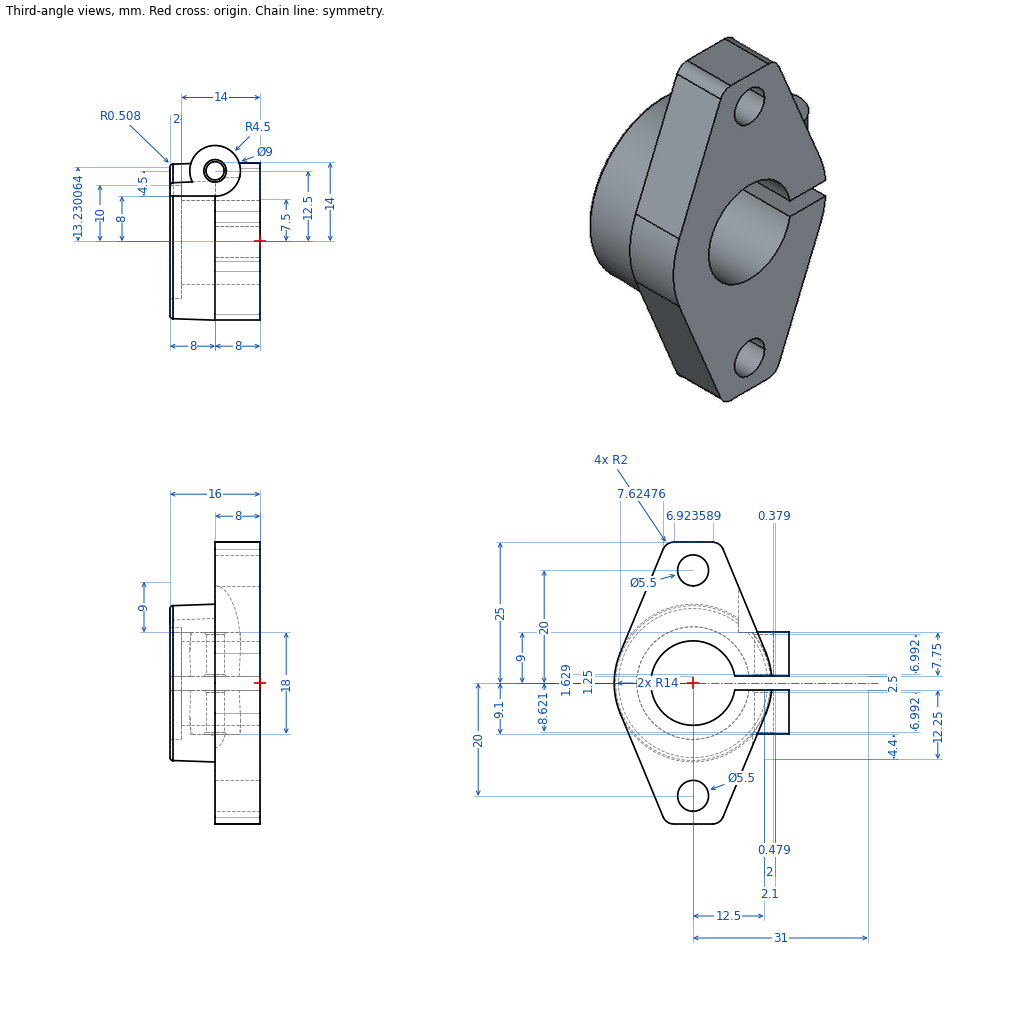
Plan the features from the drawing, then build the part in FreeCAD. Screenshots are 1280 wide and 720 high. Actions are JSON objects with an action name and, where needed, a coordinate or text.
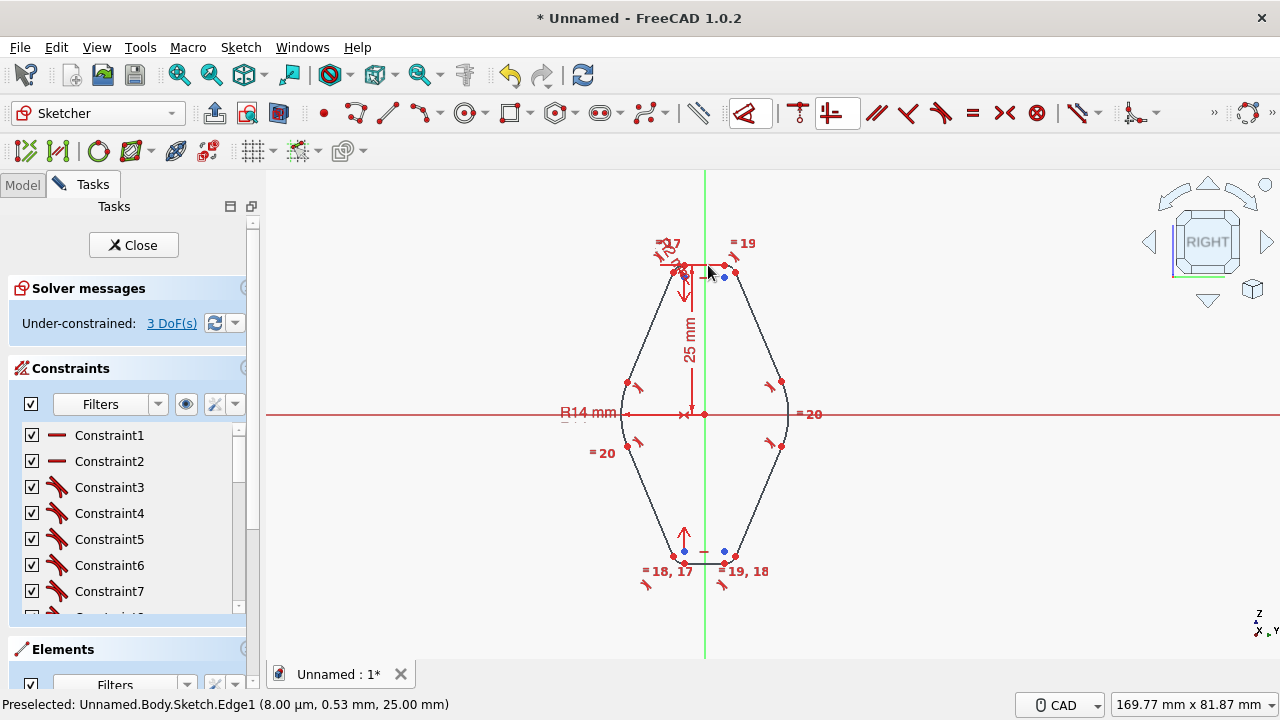
{"action": "key", "text": "l"}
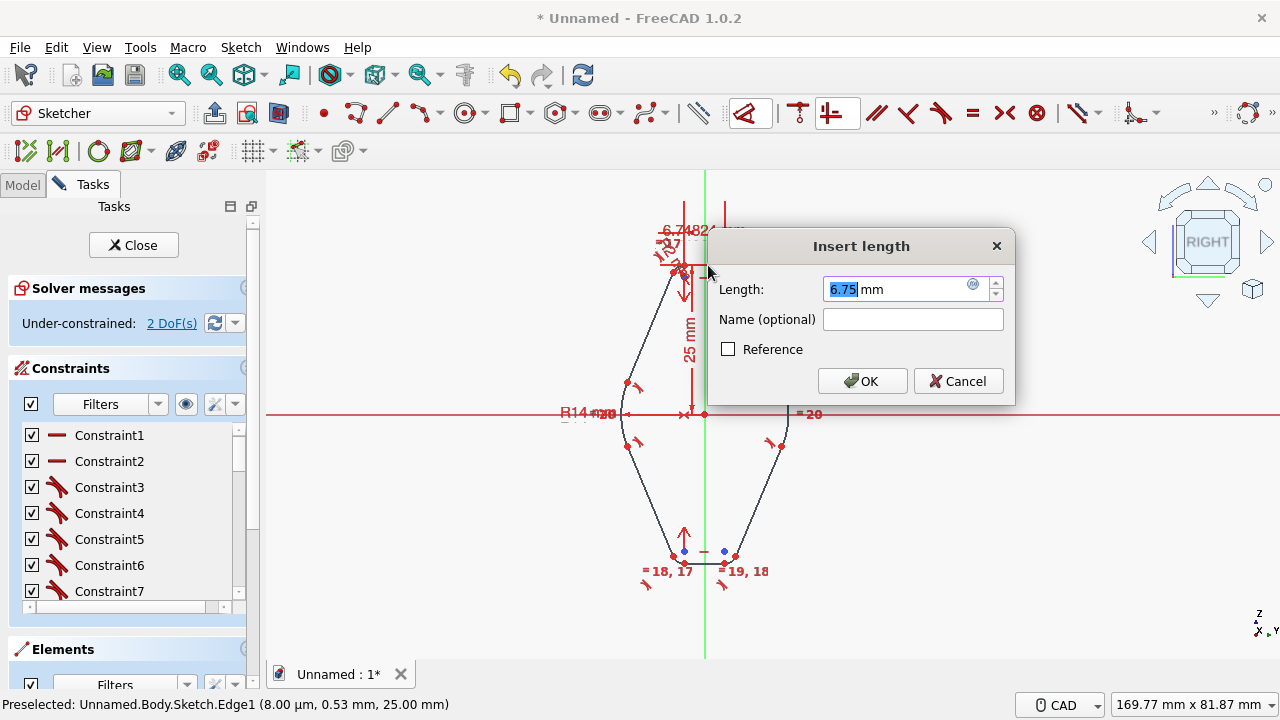
{"action": "type", "text": "6.923589"}
{"action": "key", "text": "Return"}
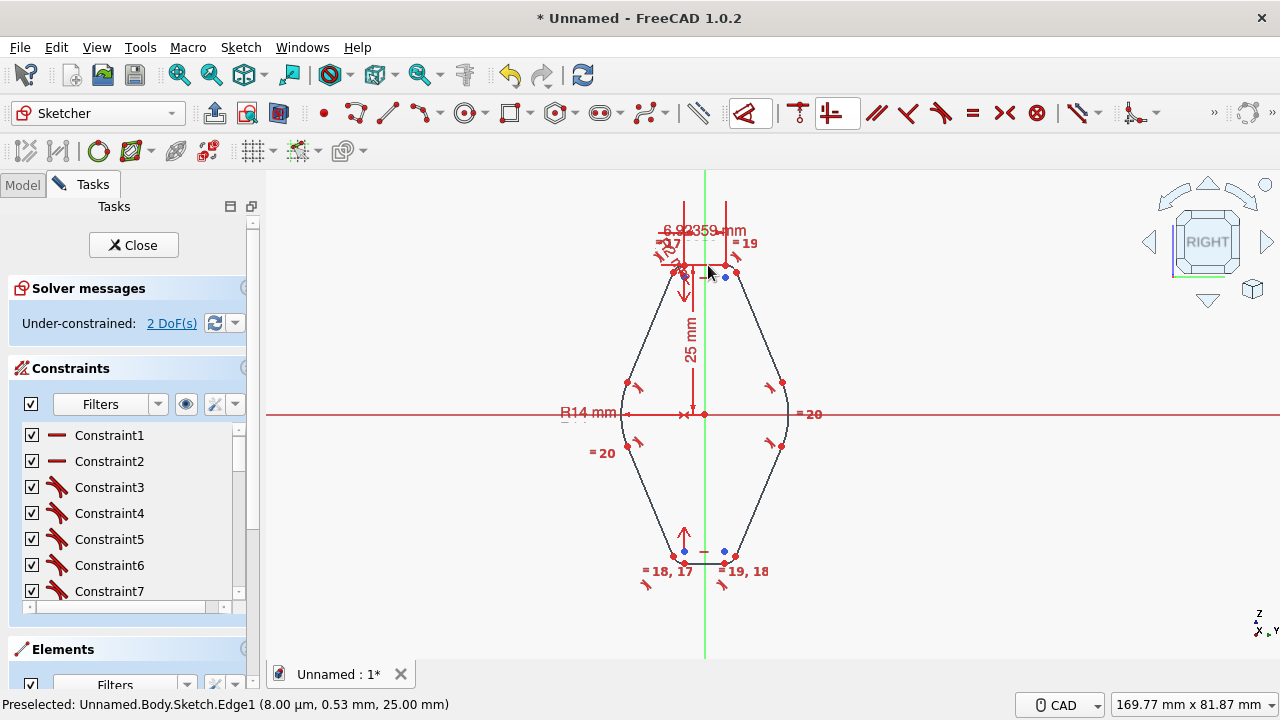
{"action": "left_click", "coordinate": [709, 564]}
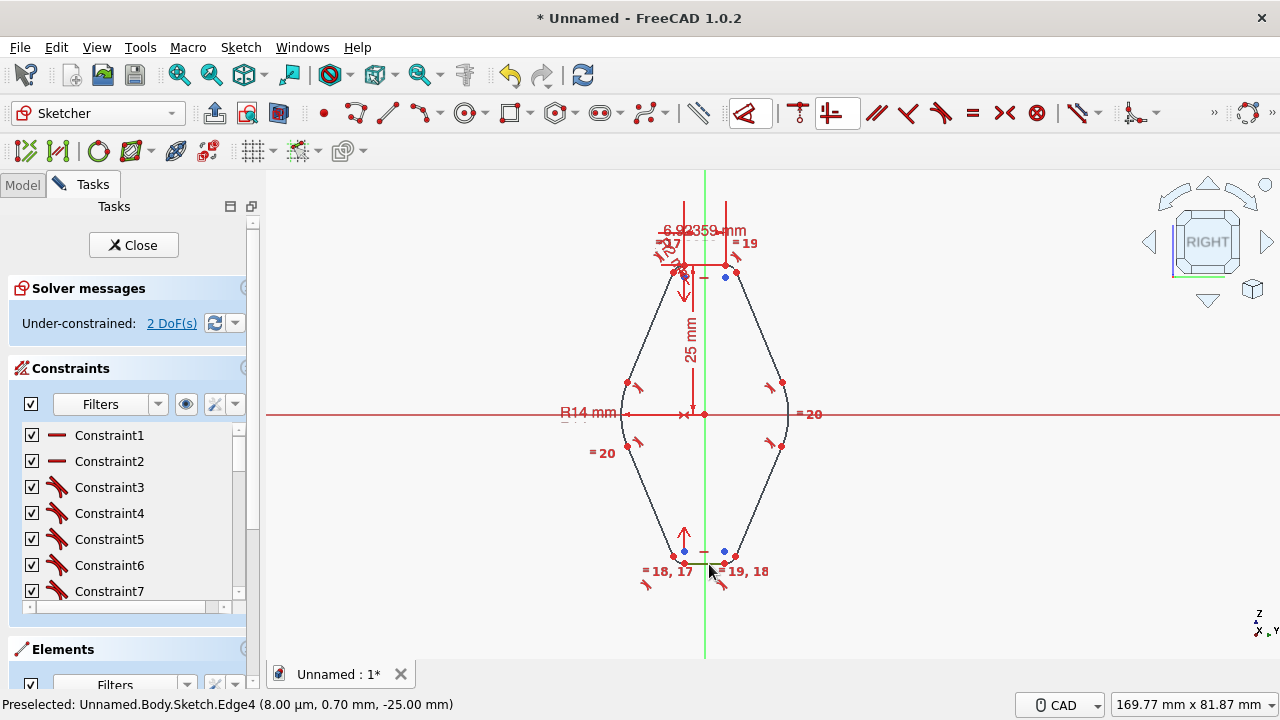
{"action": "left_click", "coordinate": [766, 114]}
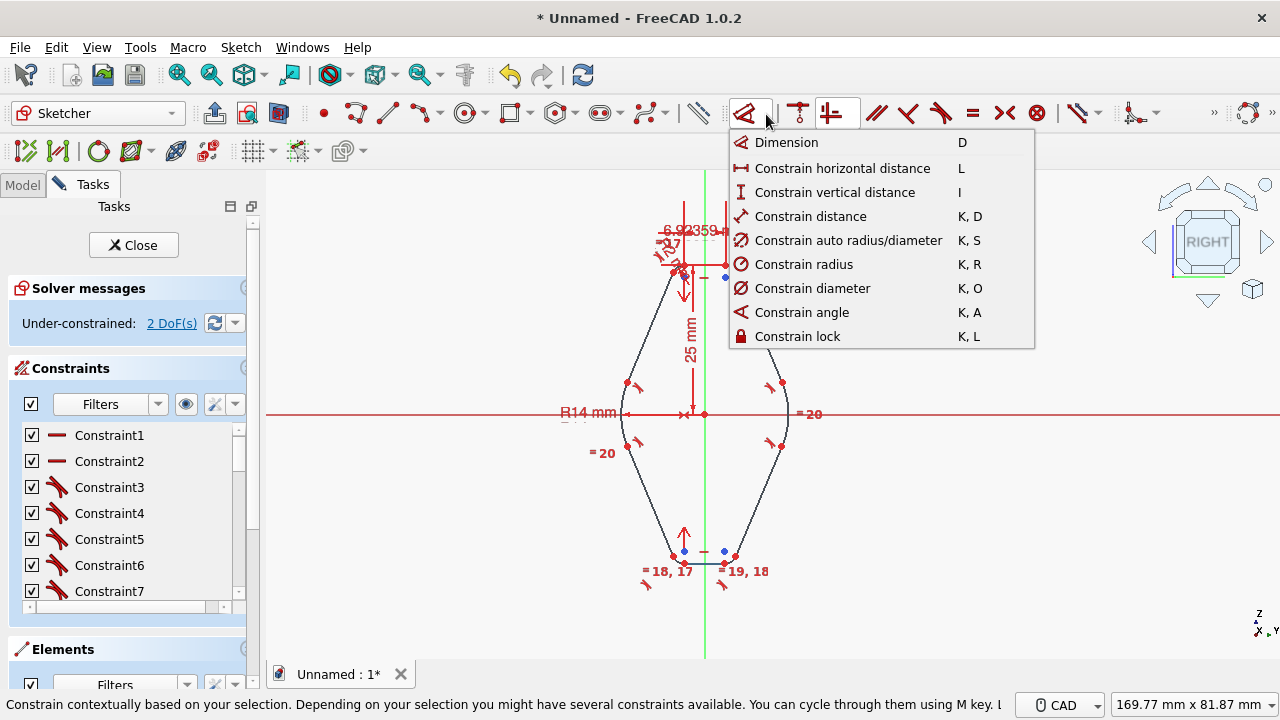
{"action": "left_click", "coordinate": [882, 168]}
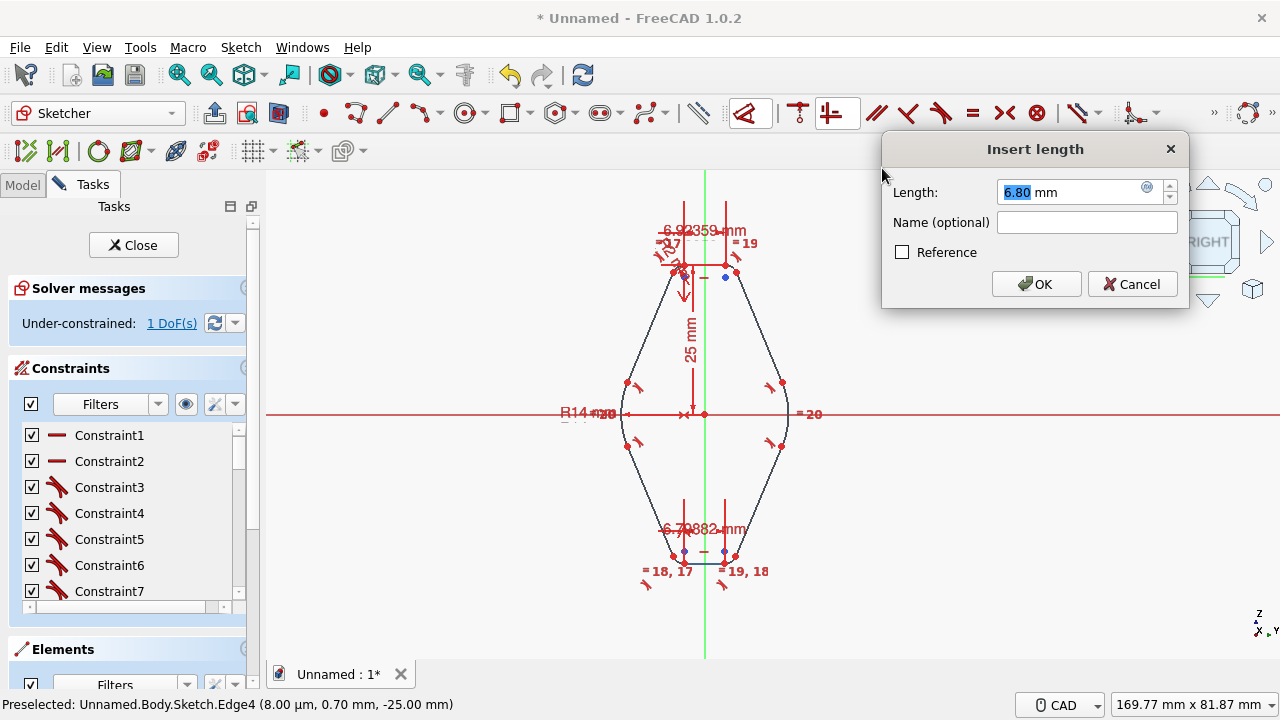
{"action": "type", "text": "6.923589"}
{"action": "key", "text": "Return"}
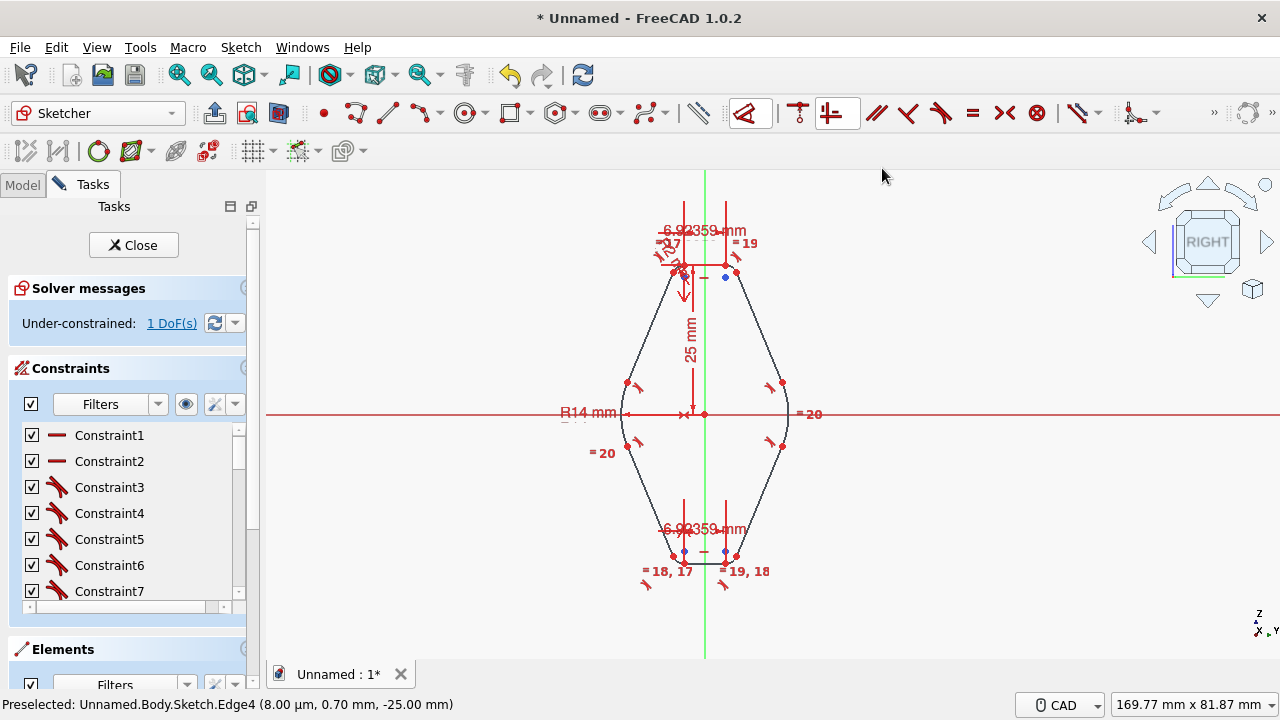
{"action": "left_click", "coordinate": [659, 306]}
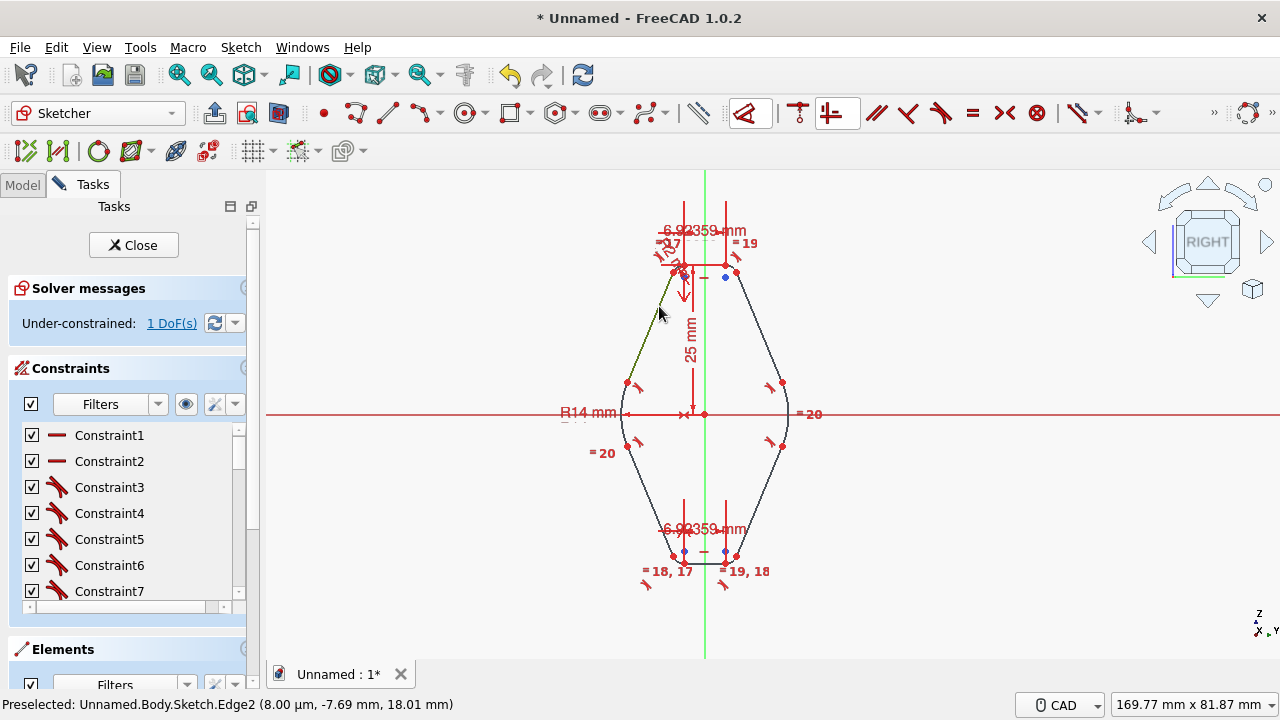
{"action": "key", "text": "l"}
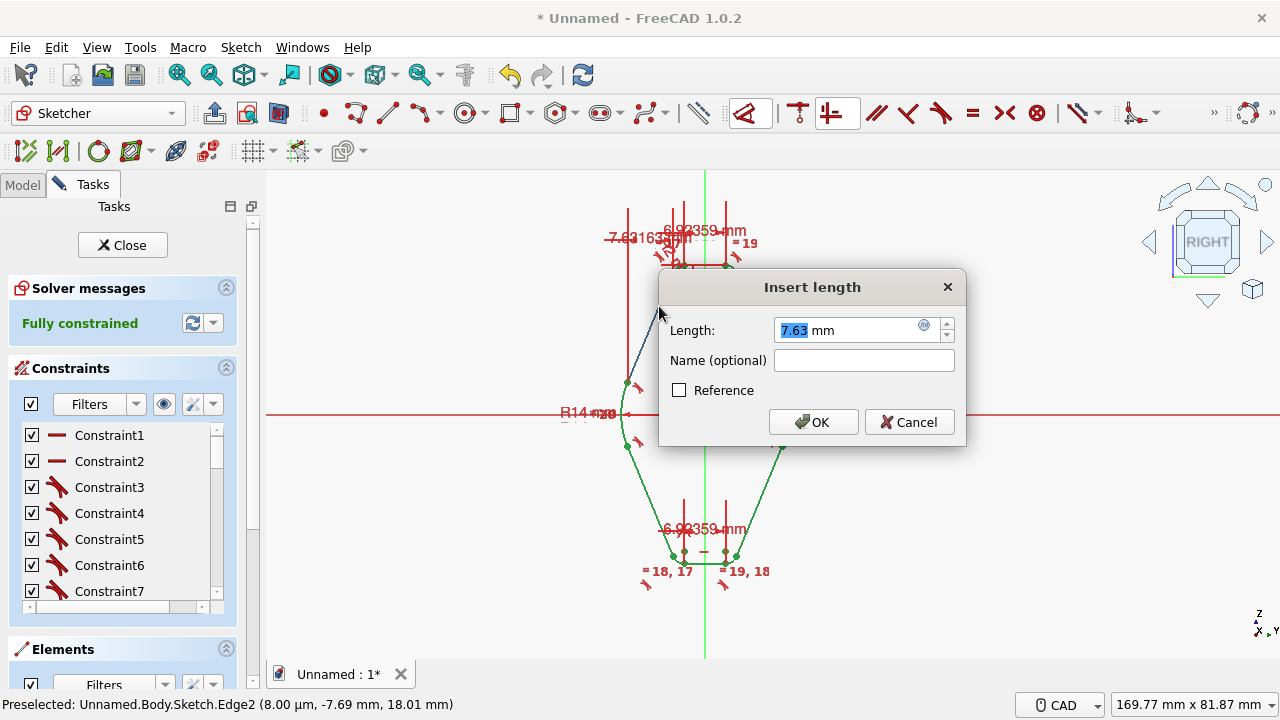
{"action": "type", "text": "7.62476"}
{"action": "key", "text": "Return"}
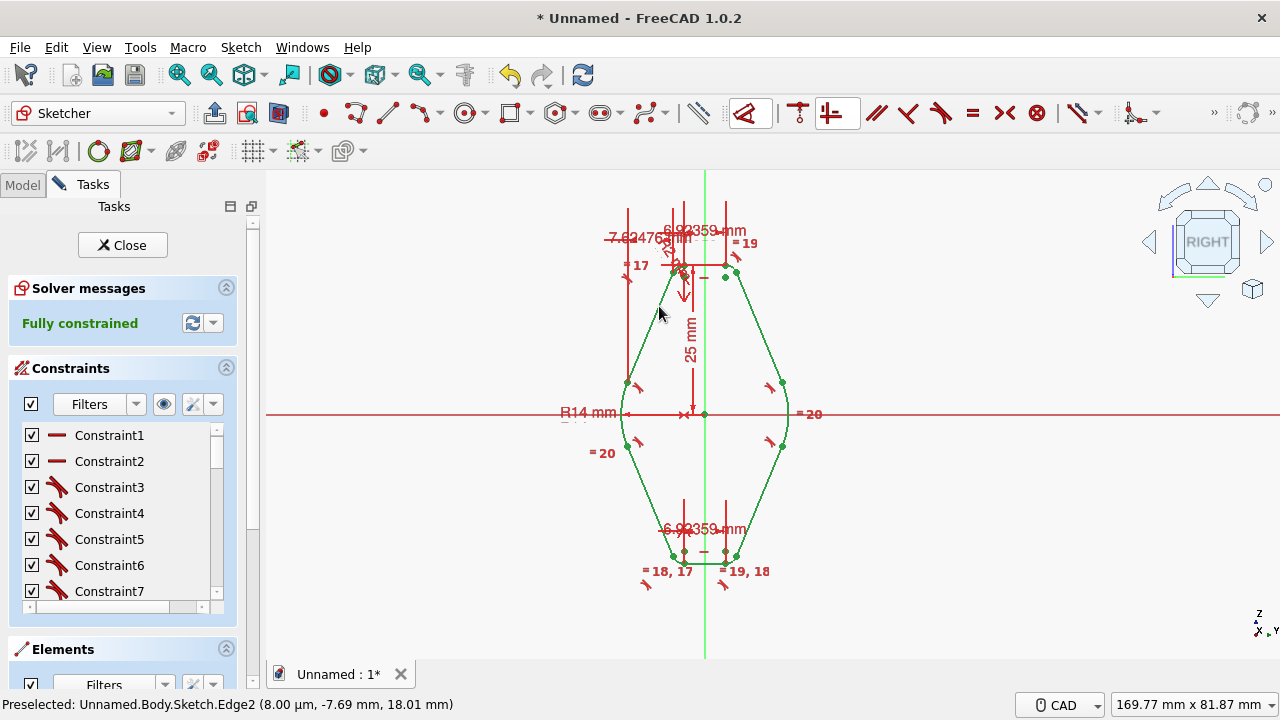
{"action": "left_click", "coordinate": [123, 245]}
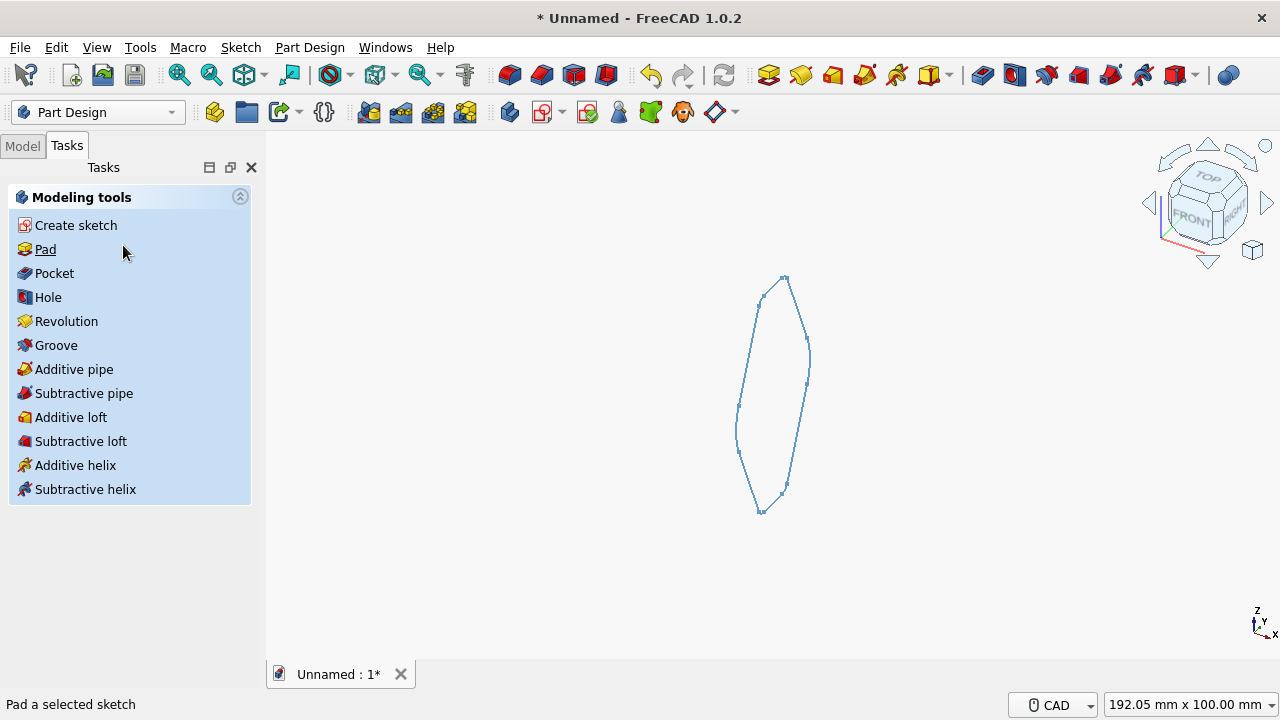
{"action": "left_click", "coordinate": [770, 76]}